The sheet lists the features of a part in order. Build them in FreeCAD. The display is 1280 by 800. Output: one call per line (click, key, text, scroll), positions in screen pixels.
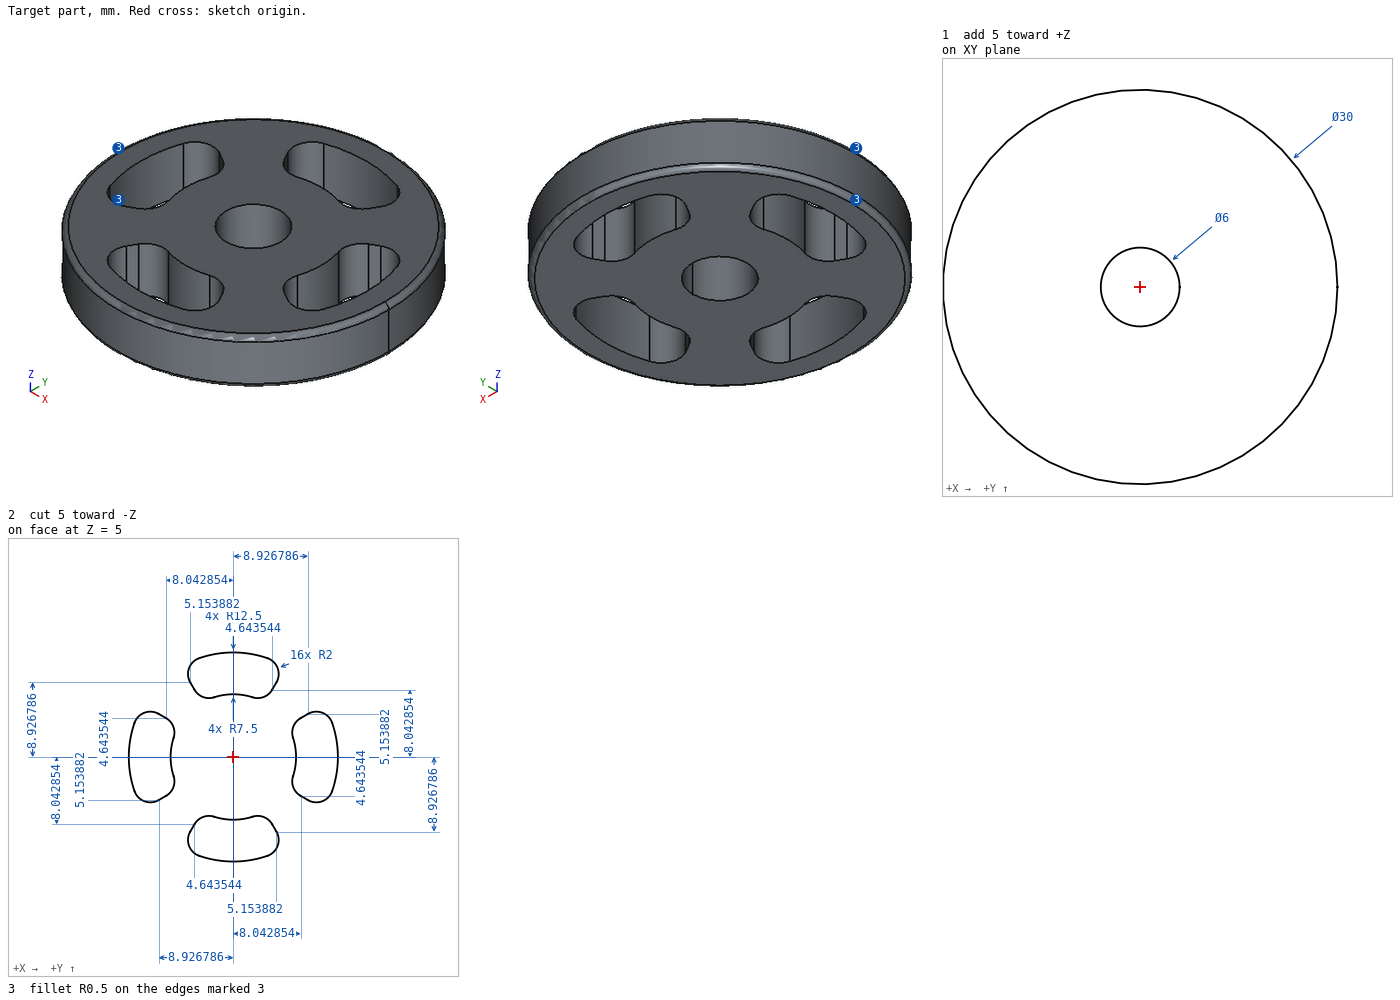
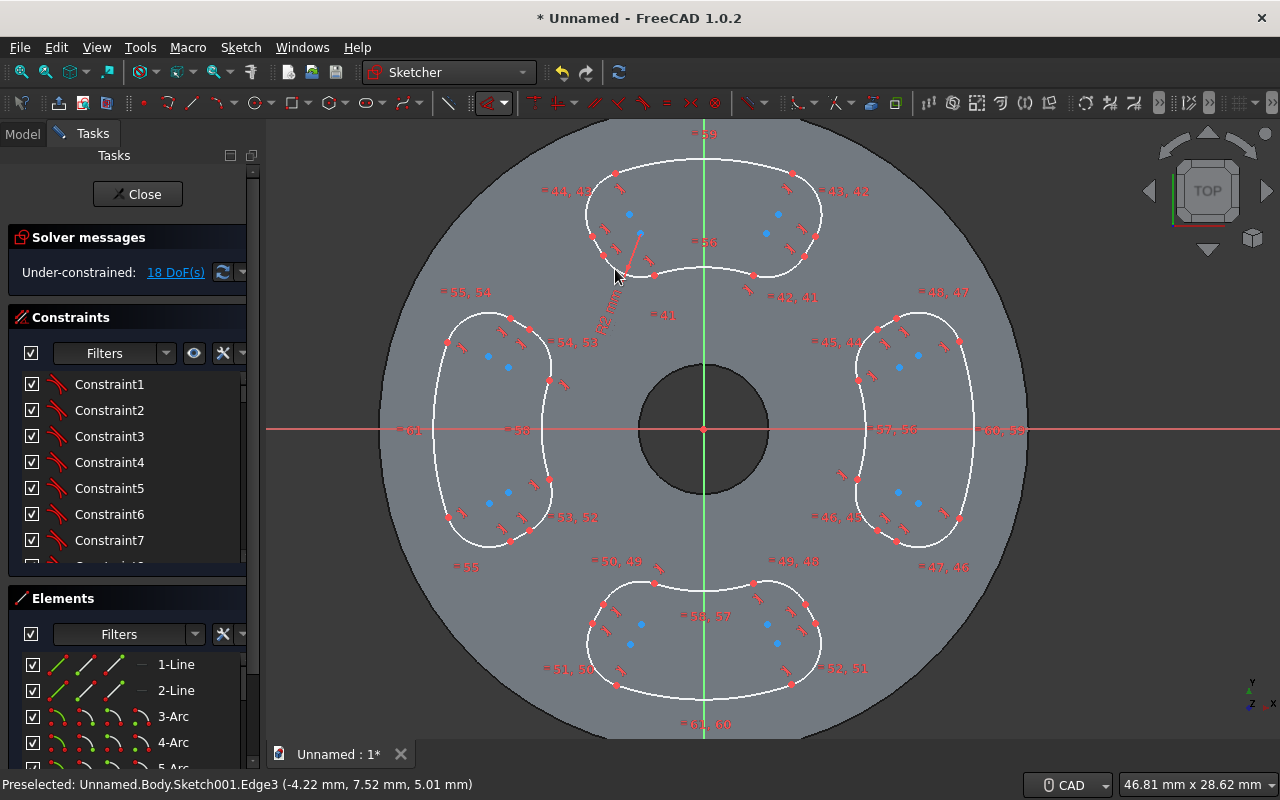
click(724, 269)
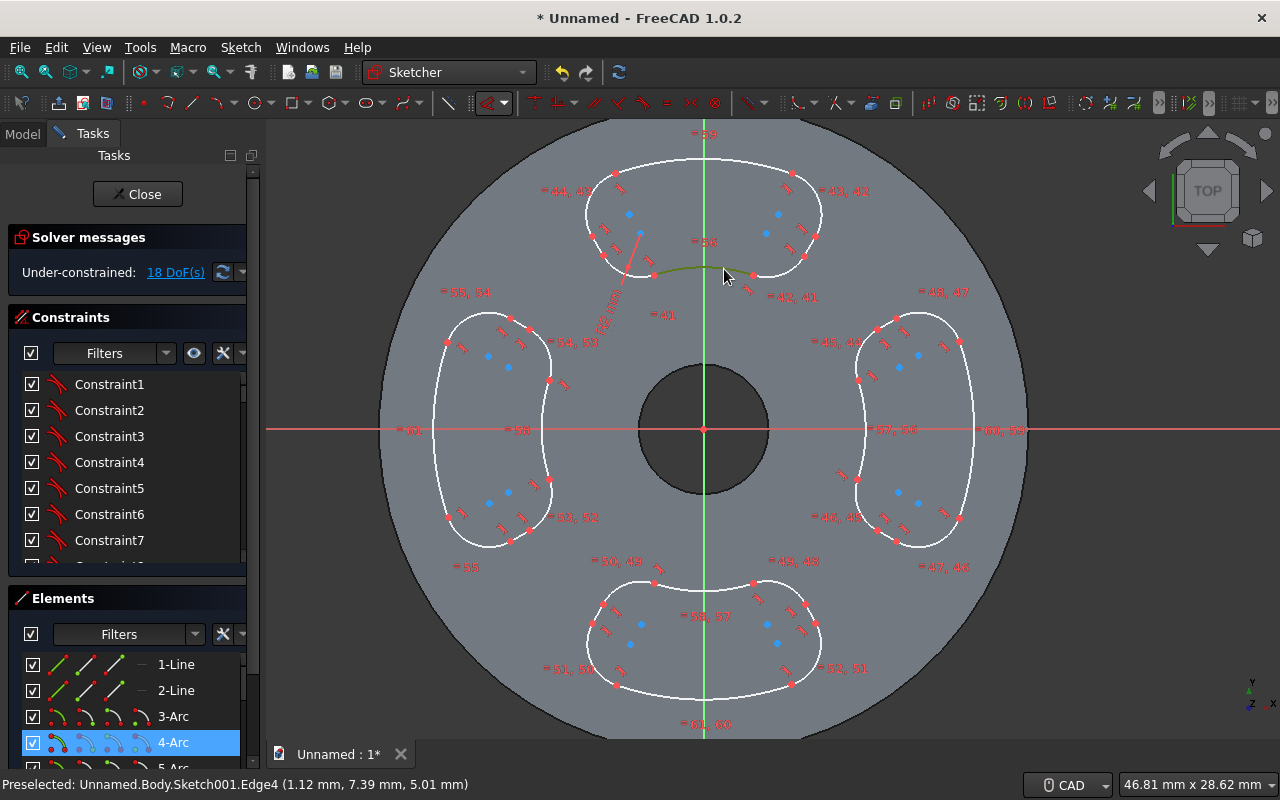
click(506, 104)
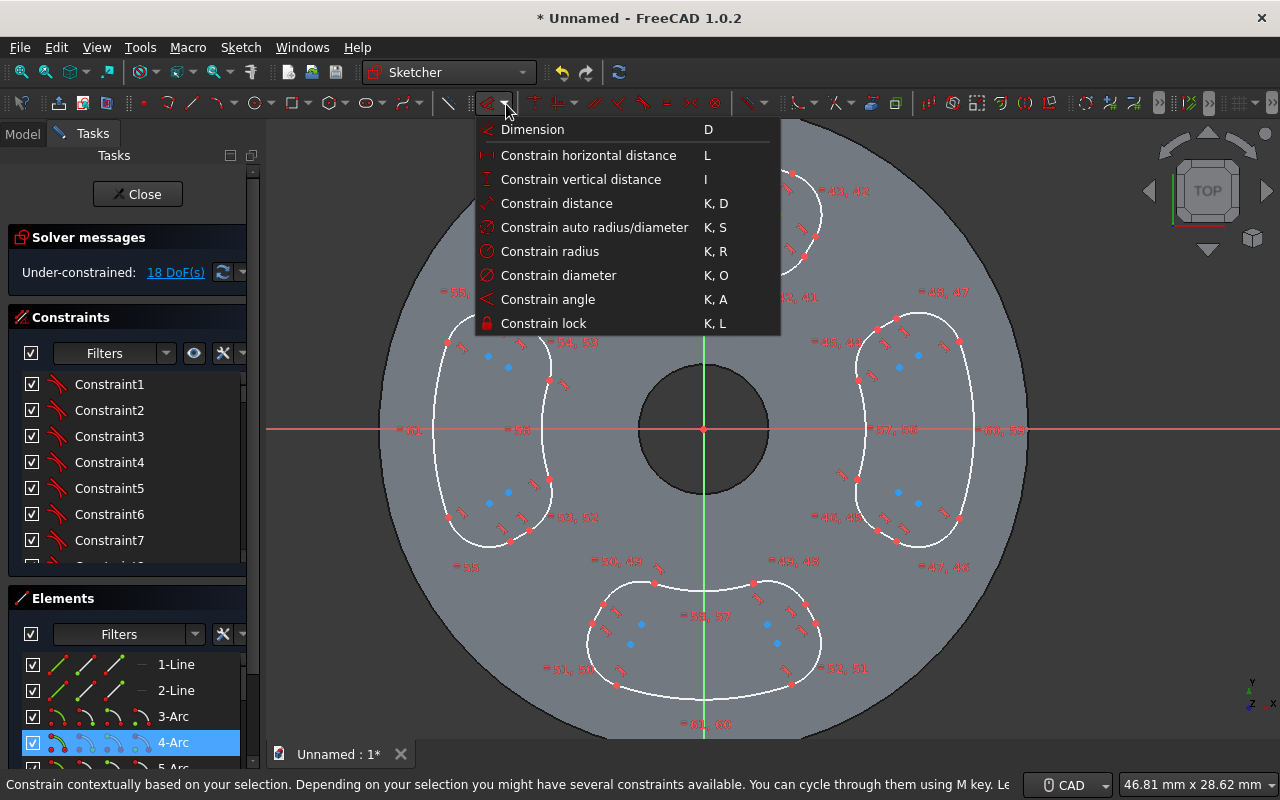
click(628, 251)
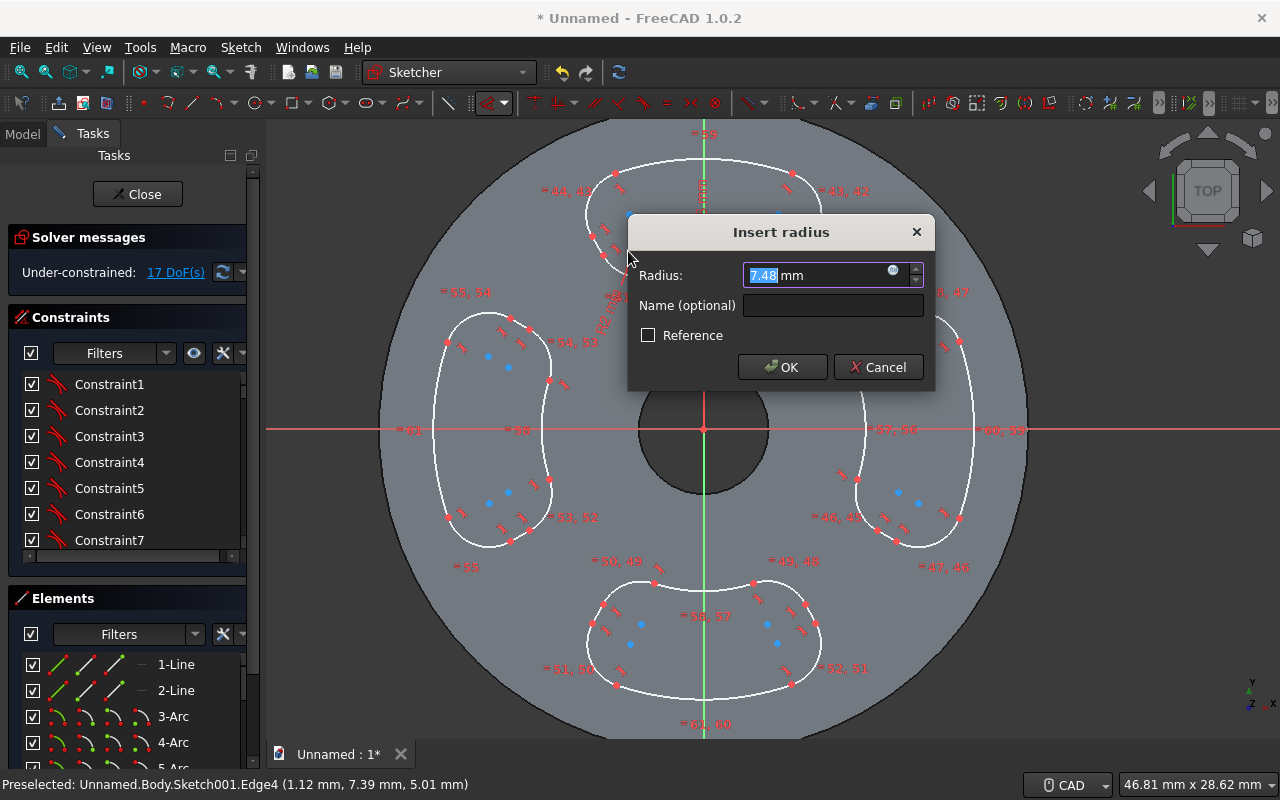
text(7.5)
key(Return)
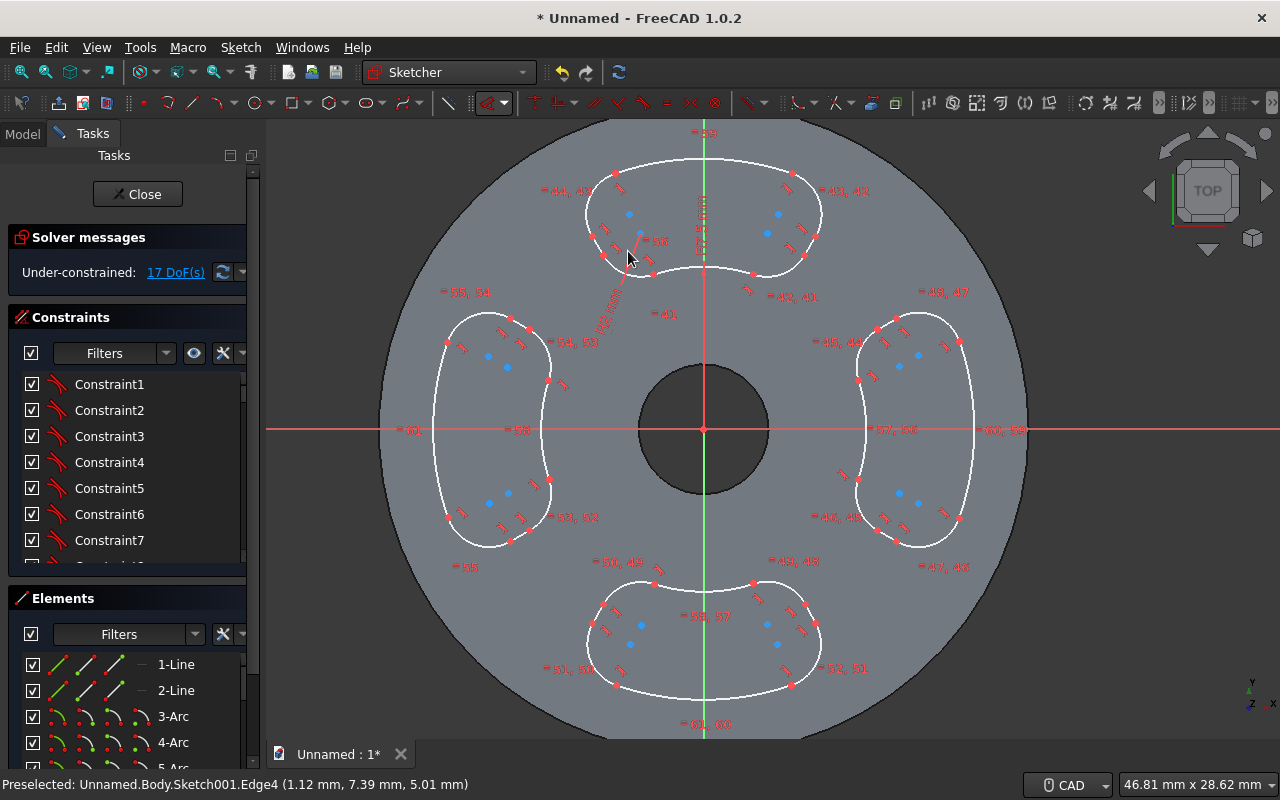
click(740, 161)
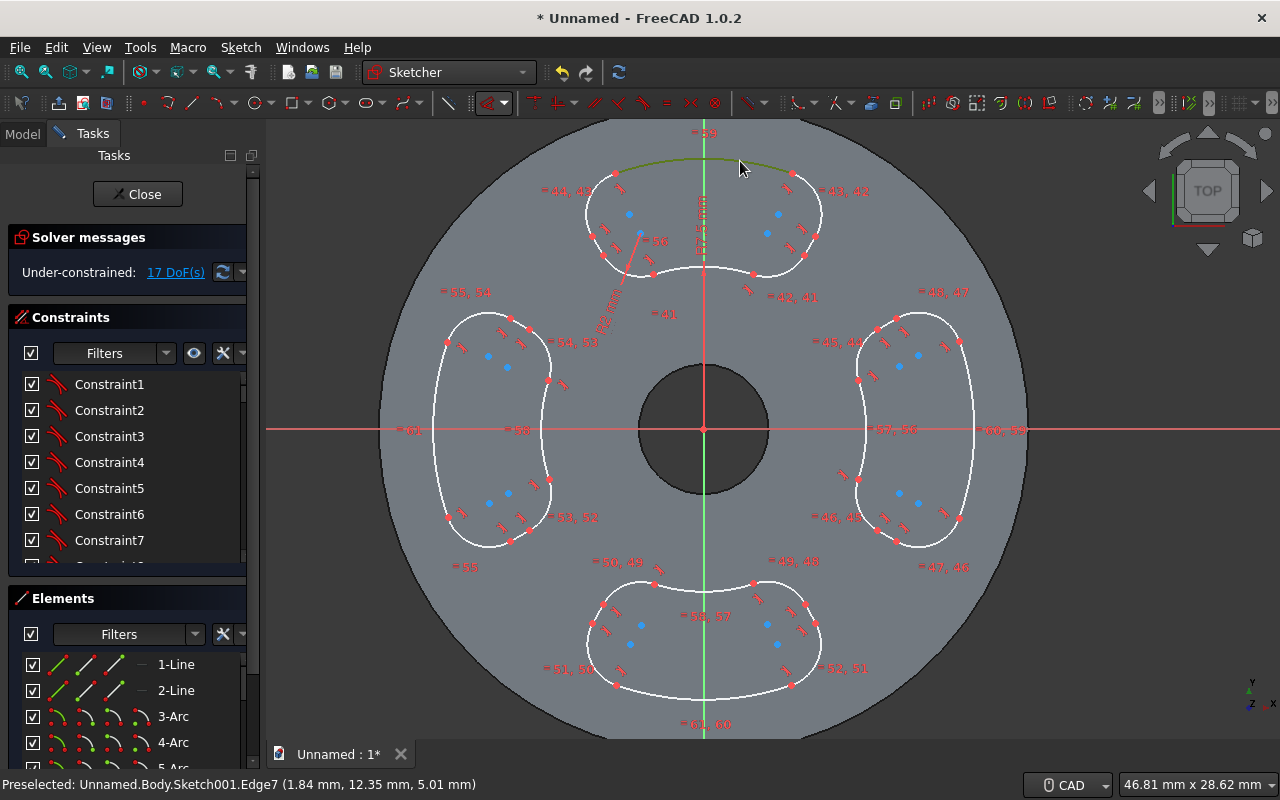
key(k)
key(r)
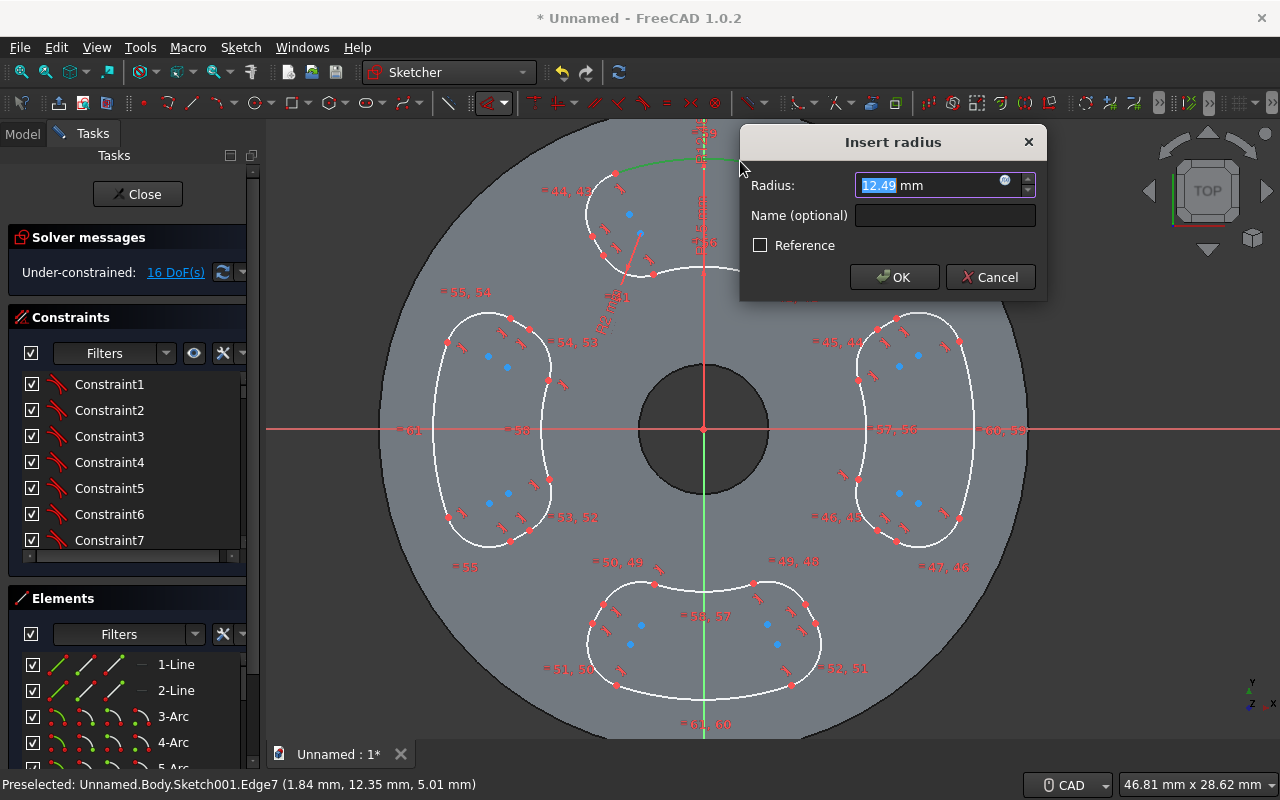
text(12.5)
key(Return)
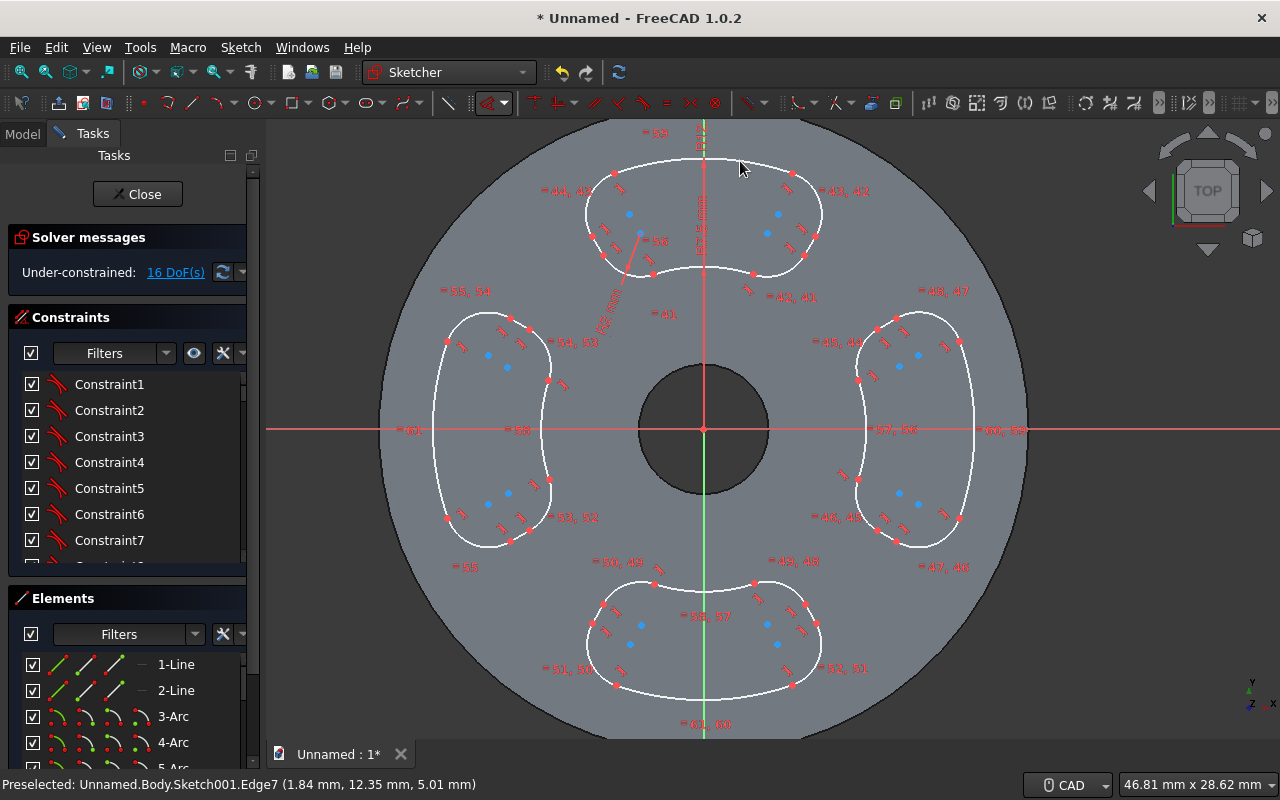
click(592, 237)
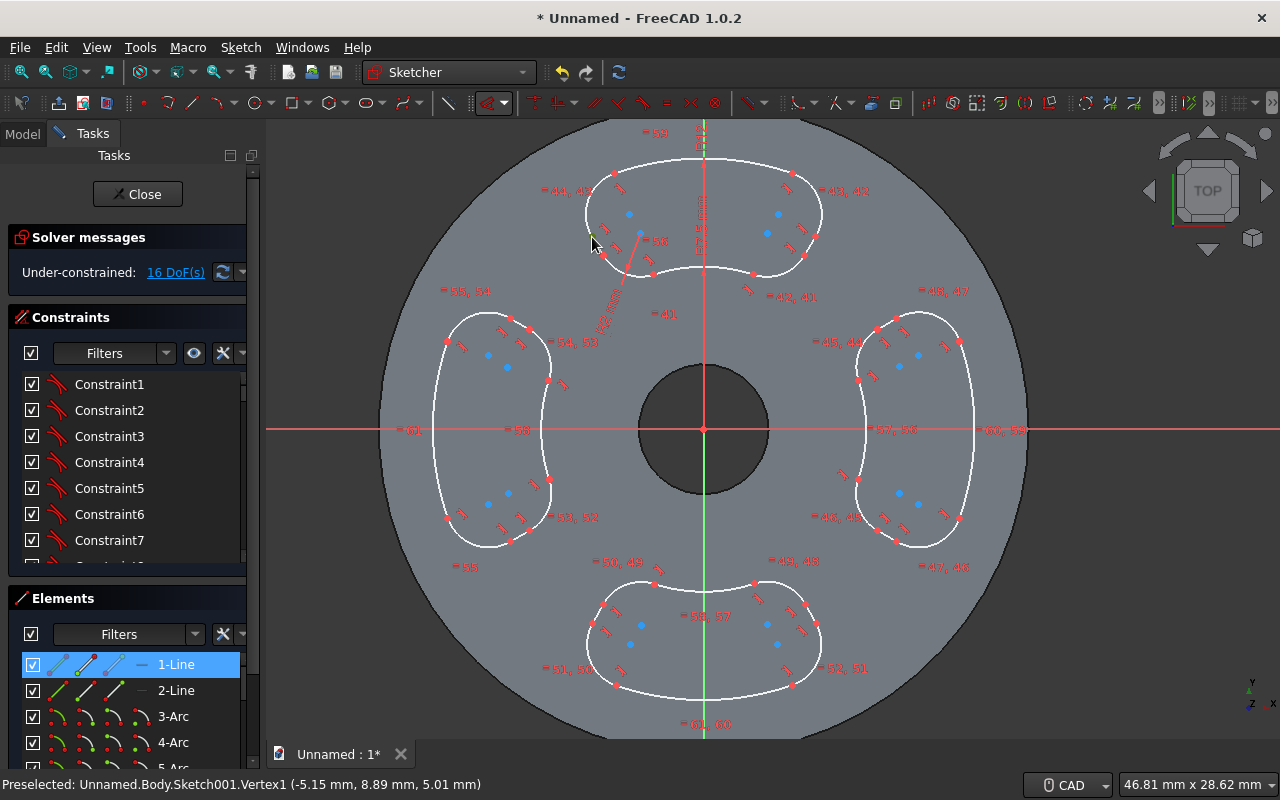
click(506, 104)